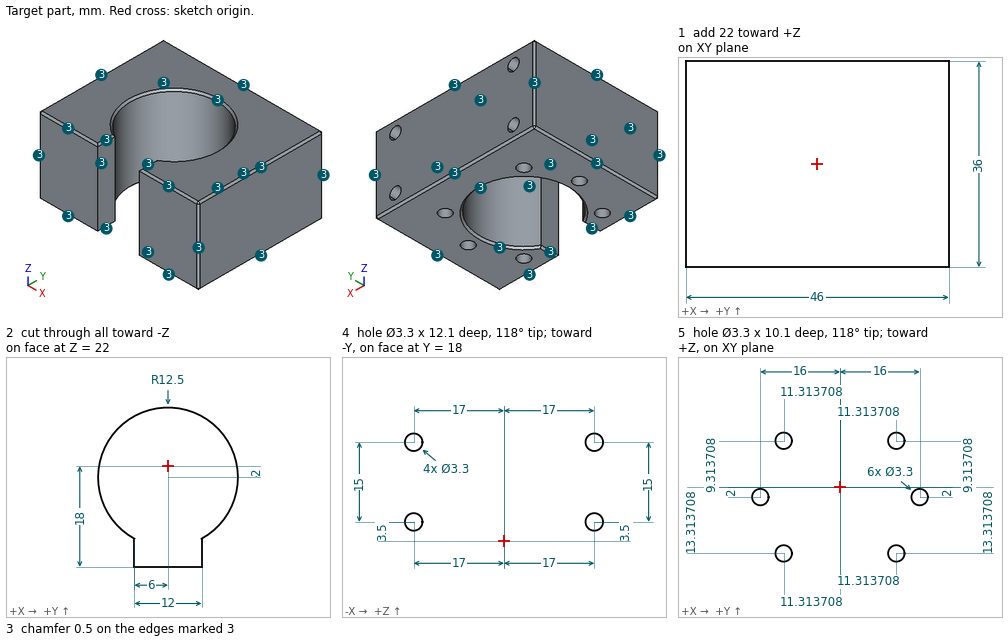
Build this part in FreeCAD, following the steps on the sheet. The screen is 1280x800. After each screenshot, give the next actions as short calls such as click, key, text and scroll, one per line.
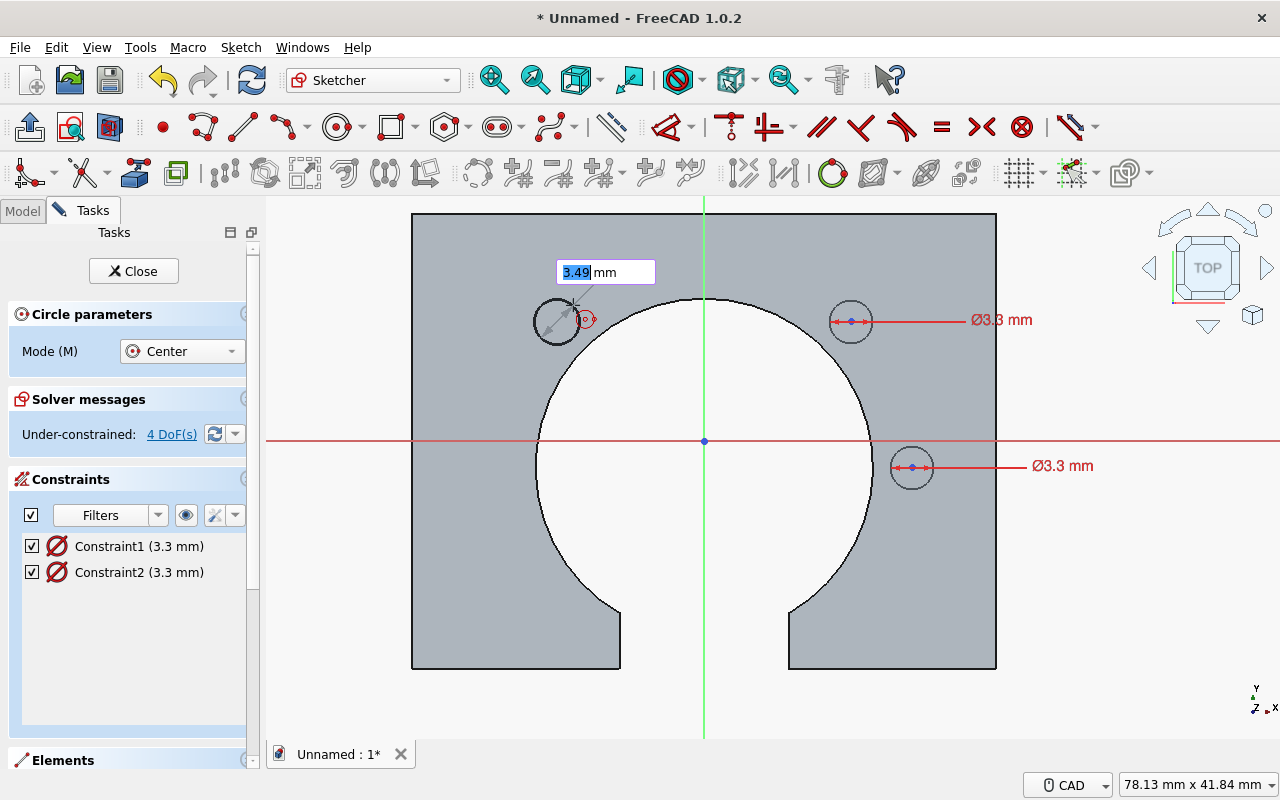
text(3.3)
key(Return)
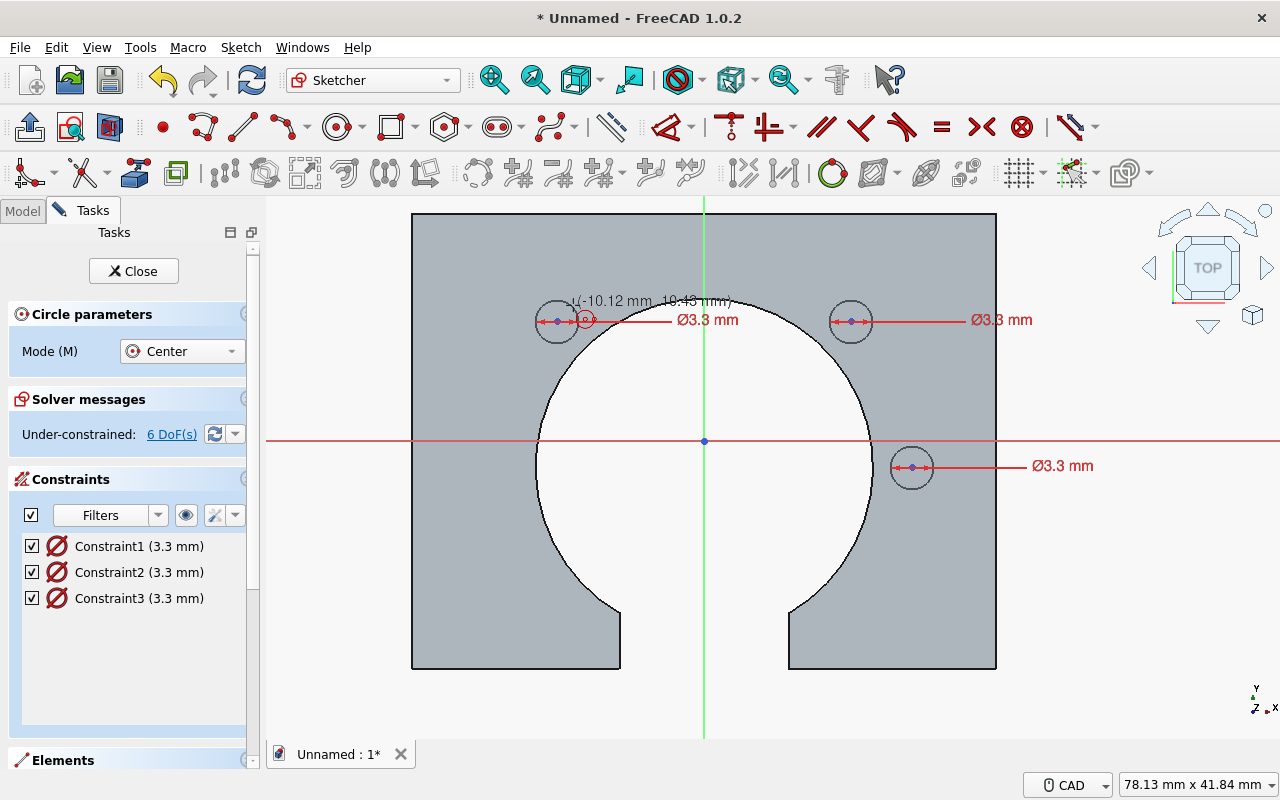
click(497, 467)
move(512, 482)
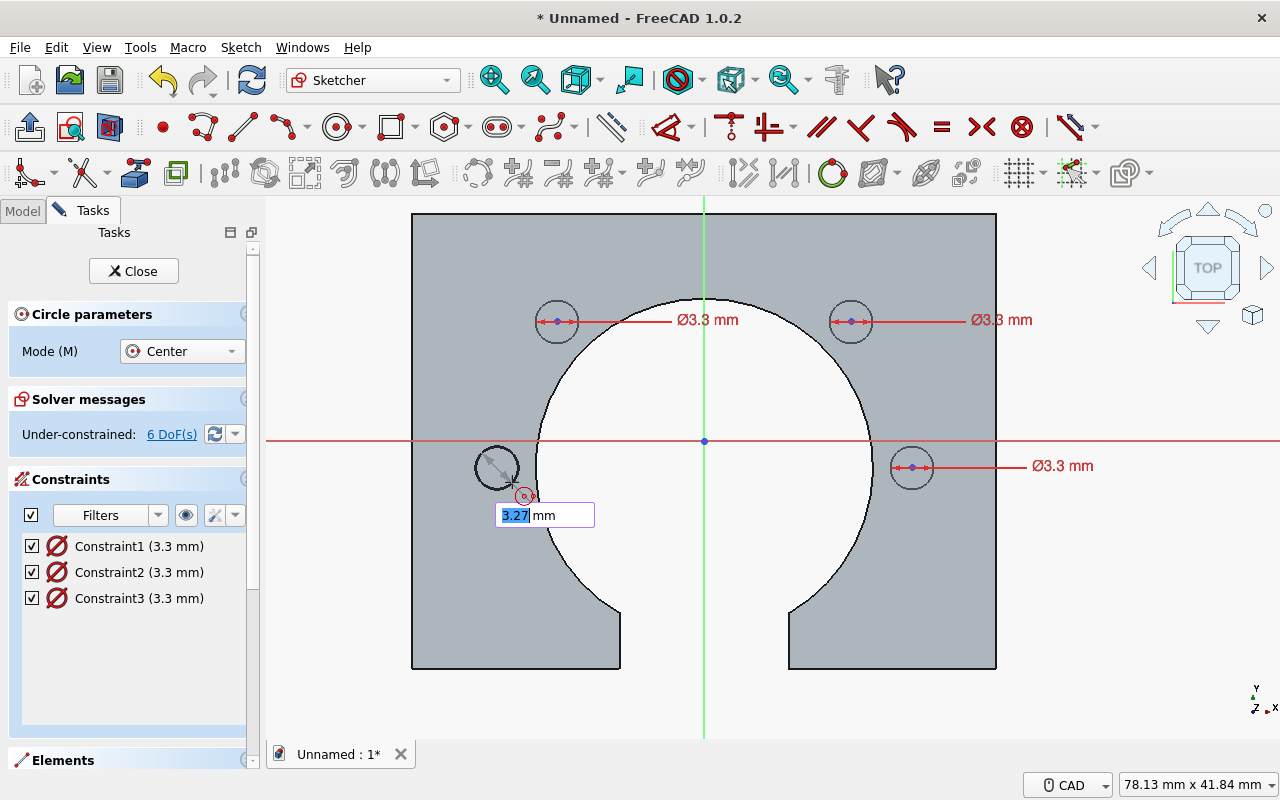
text(3.3)
key(Return)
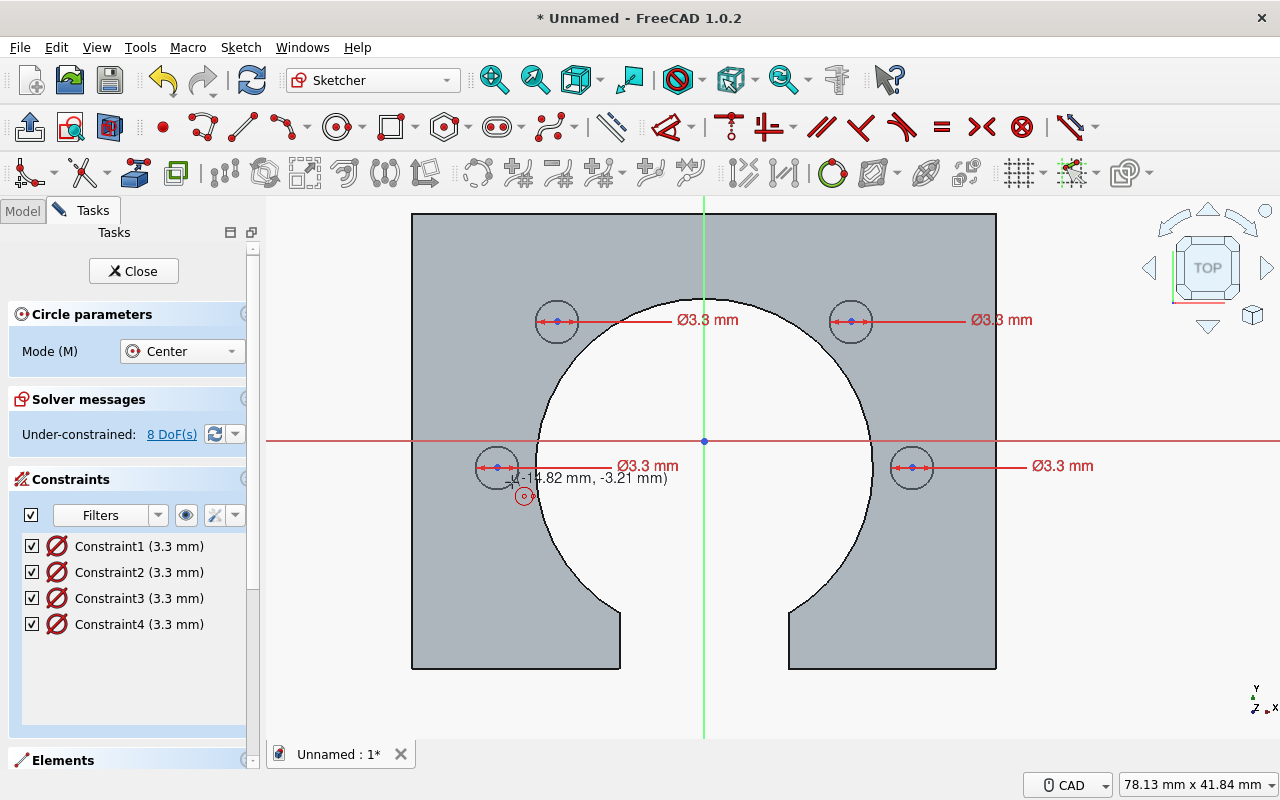
click(851, 614)
move(866, 599)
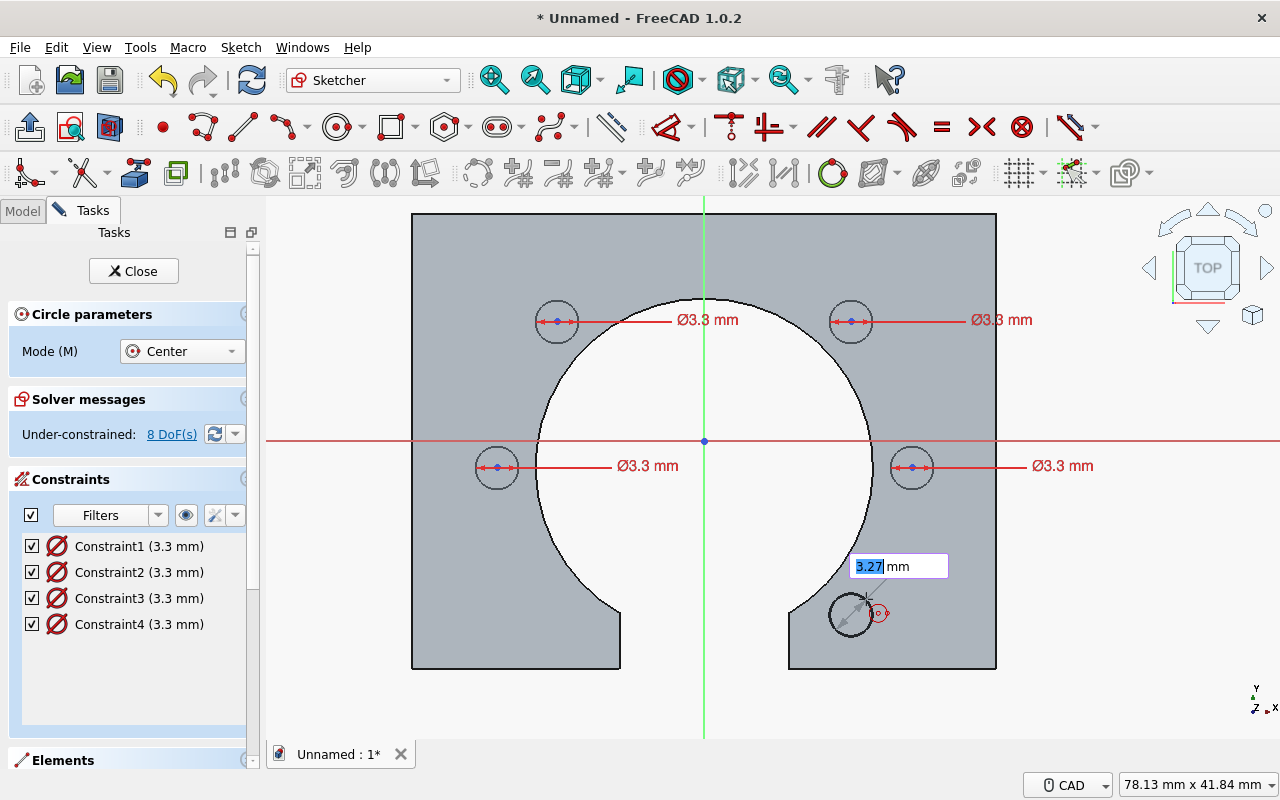
text(3.3)
key(Return)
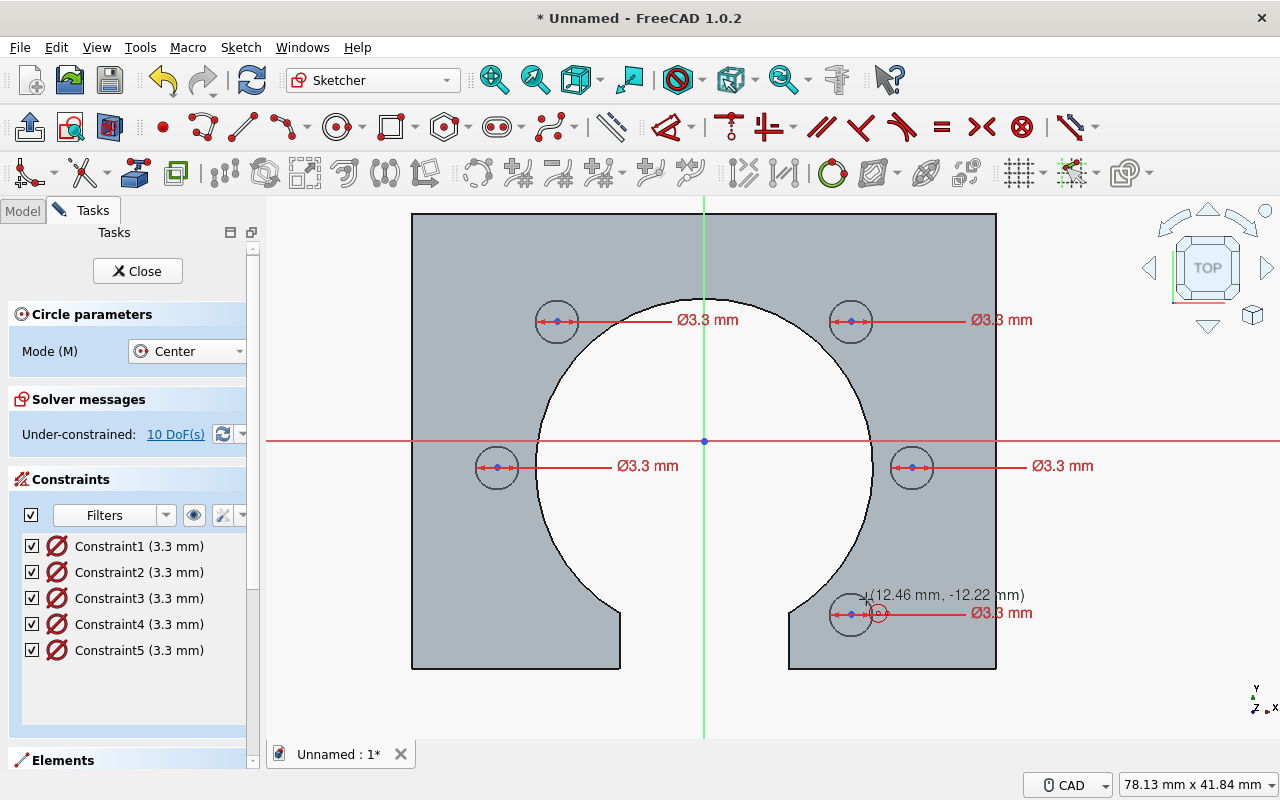
click(557, 614)
move(573, 599)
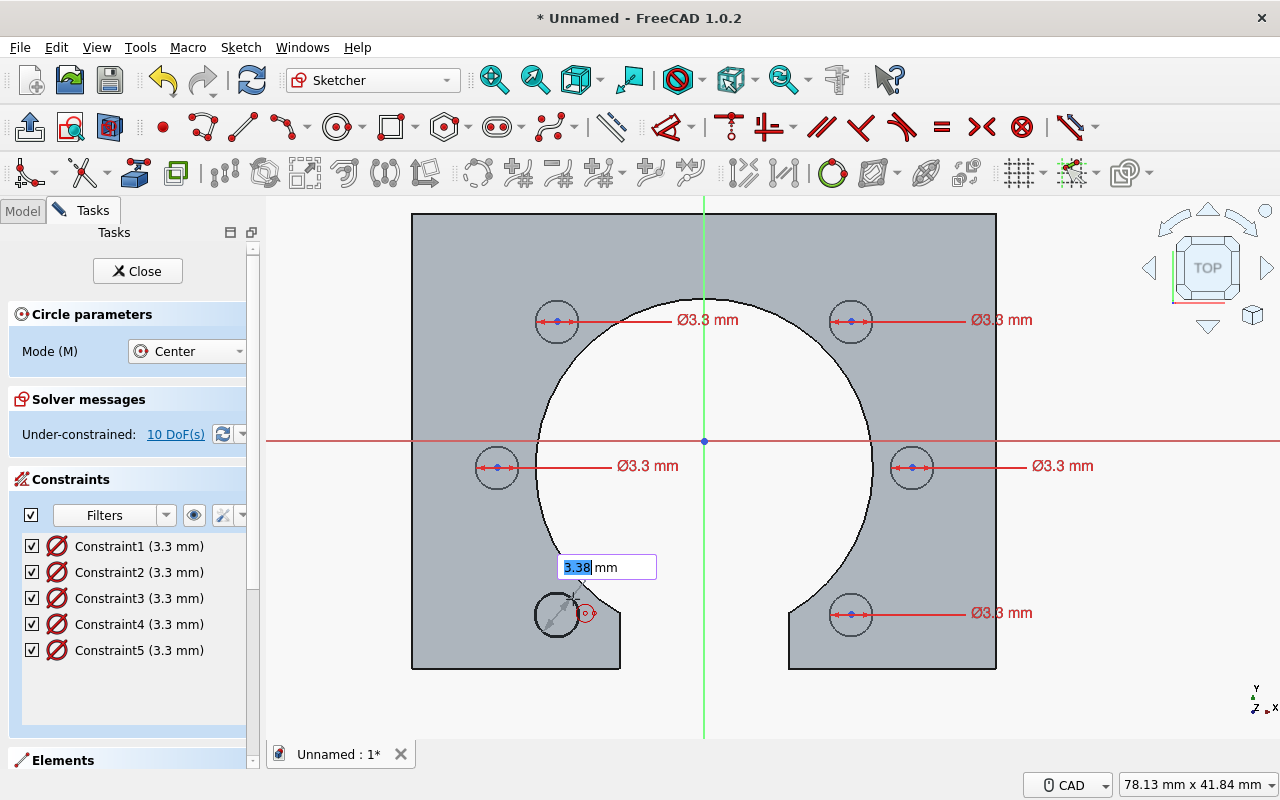
text(3.3)
key(Return)
key(Escape)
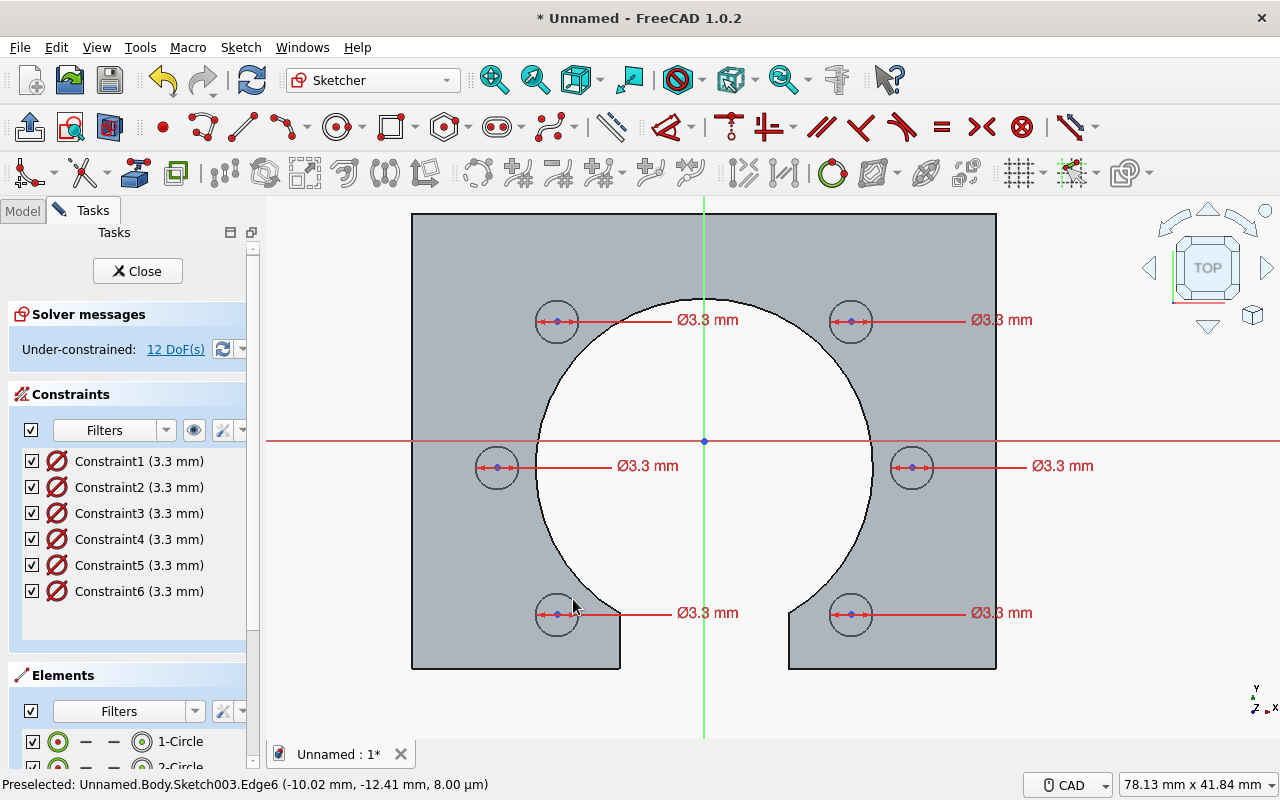
click(666, 128)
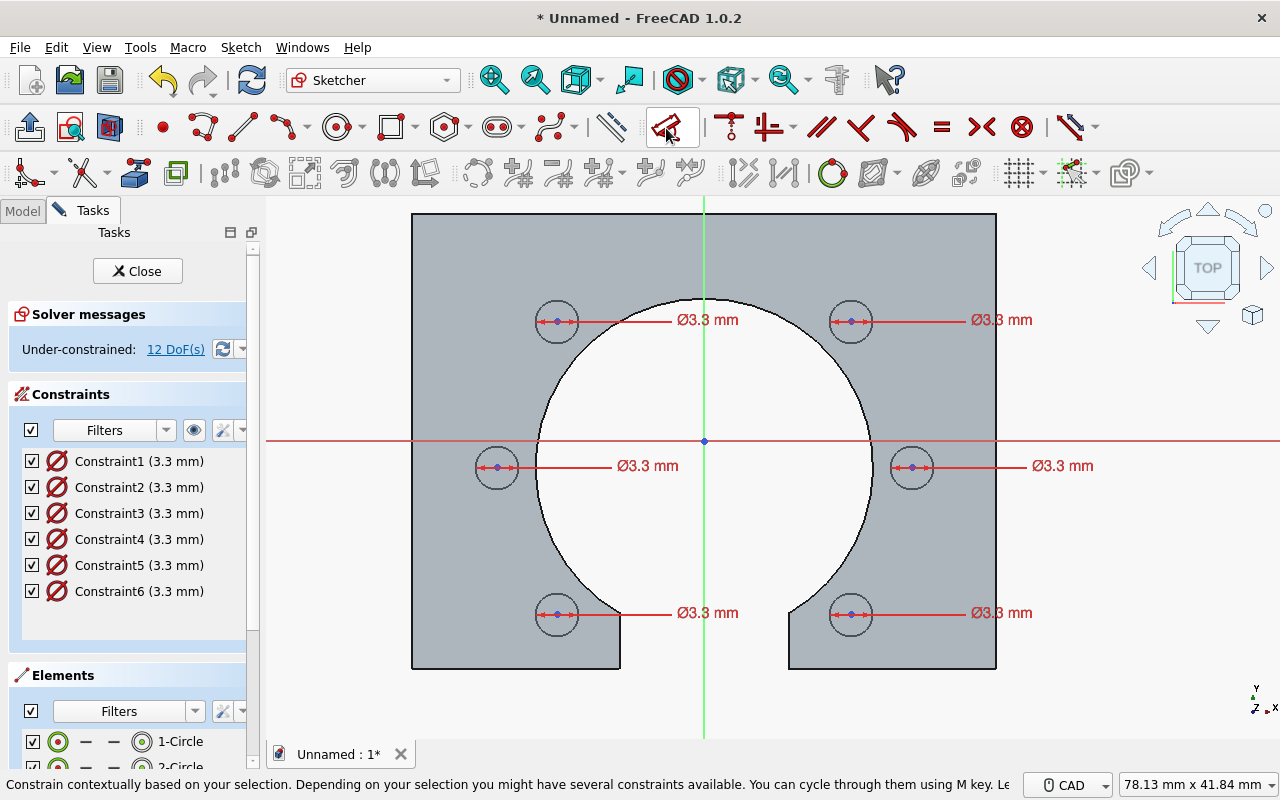
scroll(912, 468, up, 3)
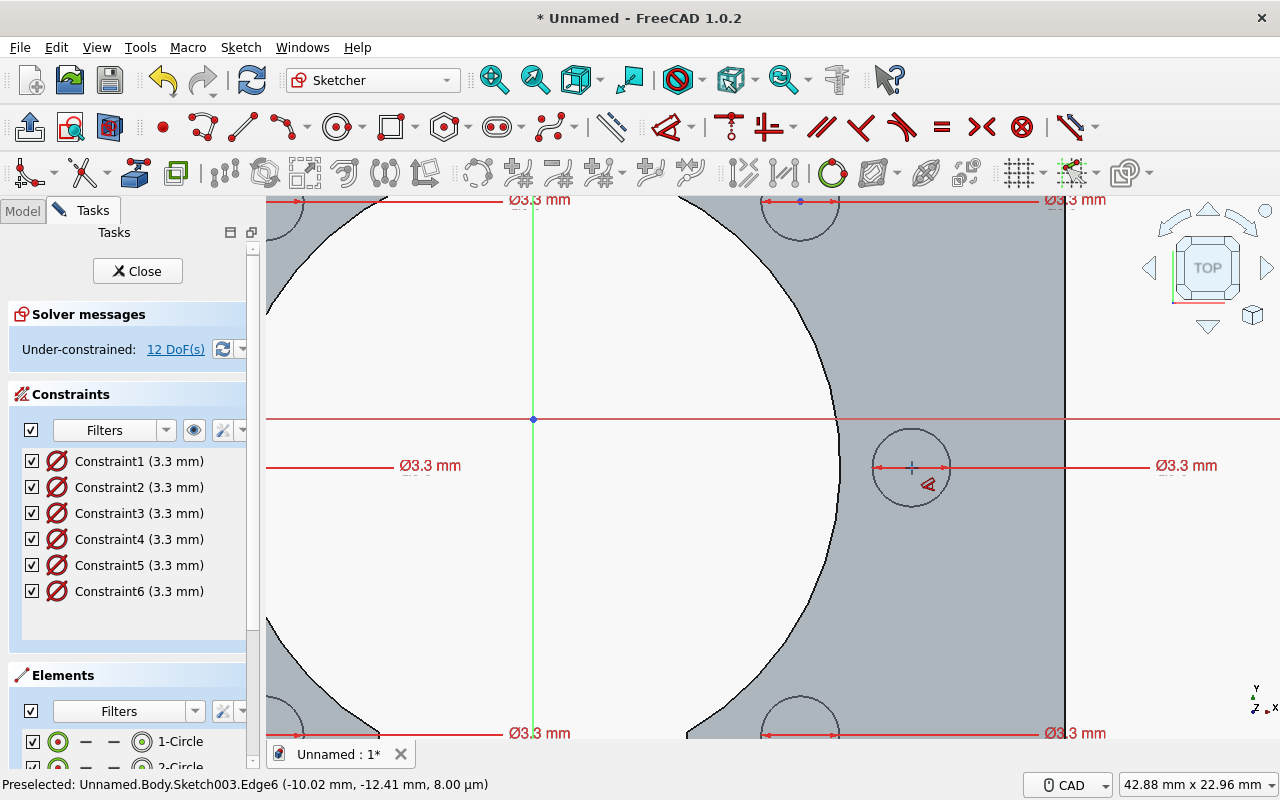
click(911, 468)
click(499, 443)